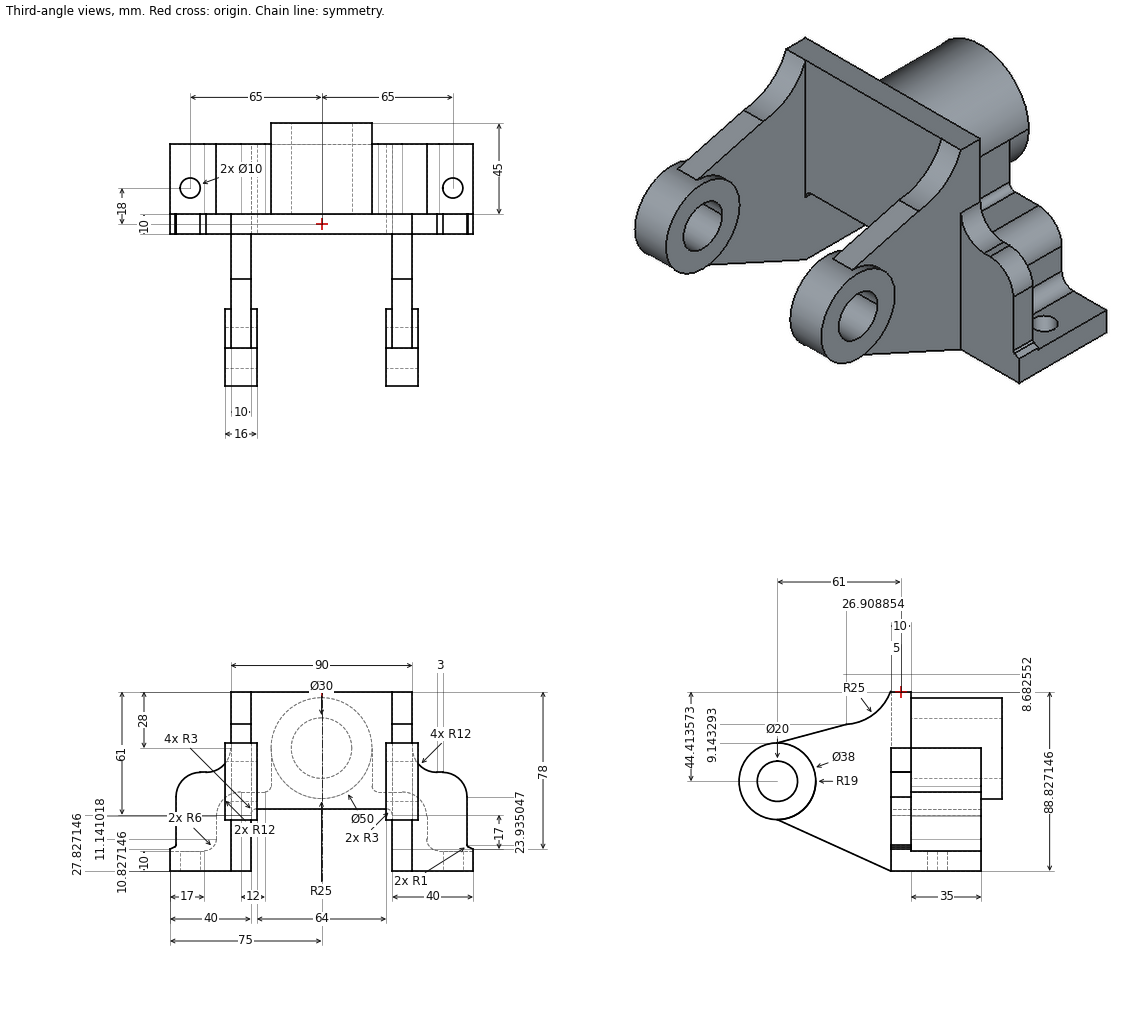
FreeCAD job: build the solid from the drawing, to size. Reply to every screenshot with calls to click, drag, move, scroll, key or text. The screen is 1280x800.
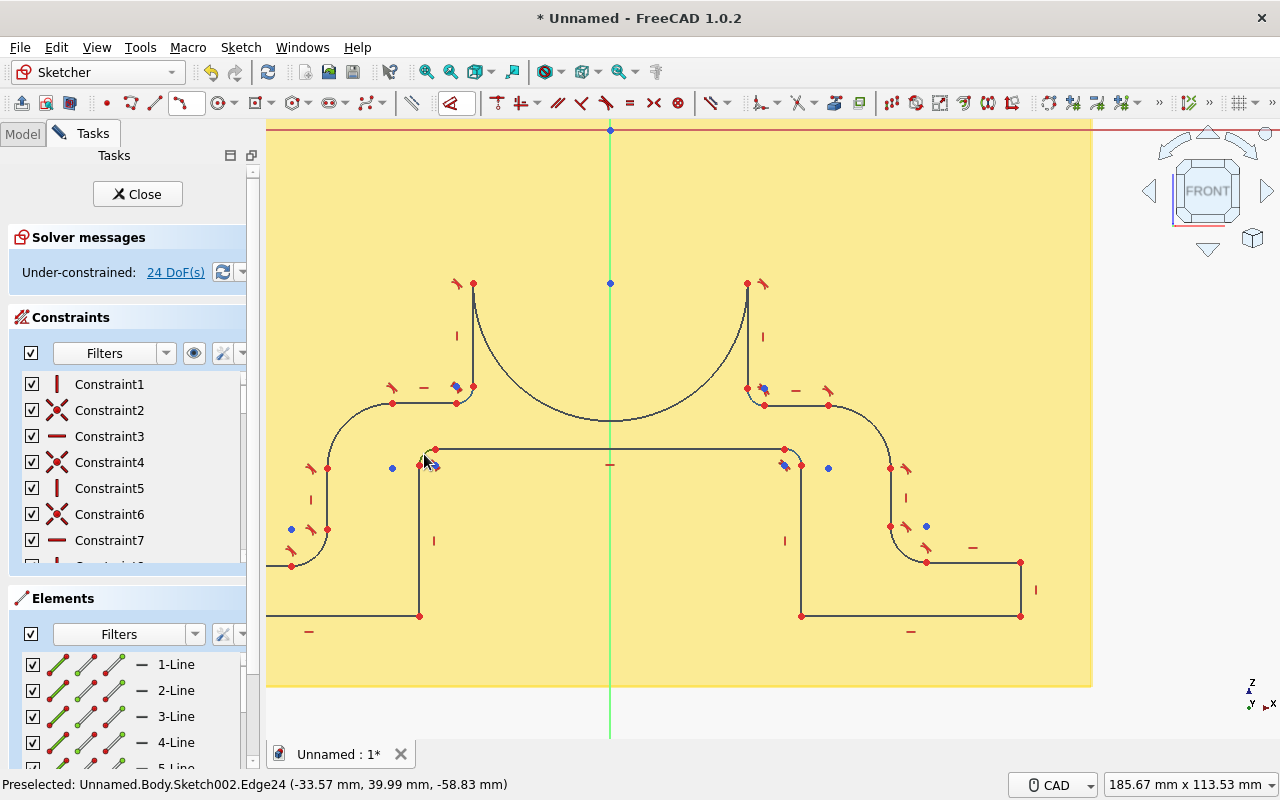
key(e)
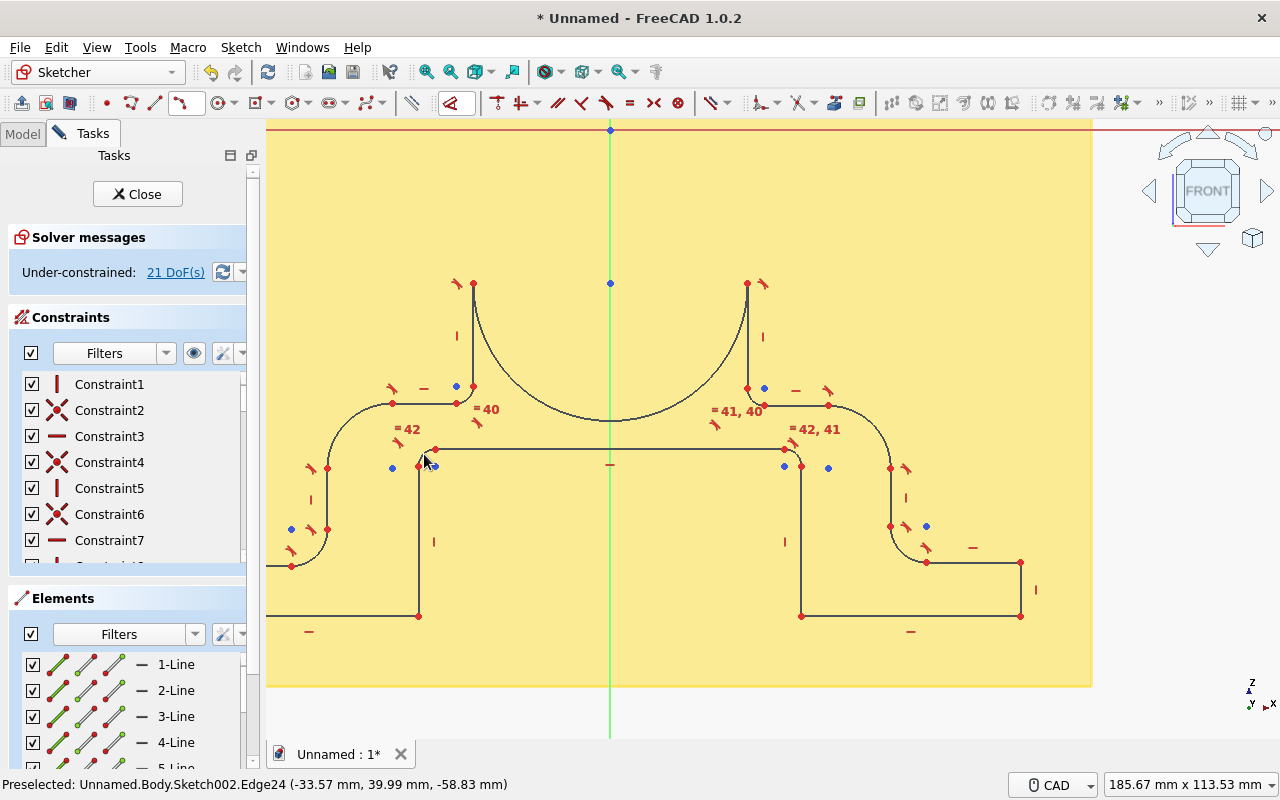
click(363, 411)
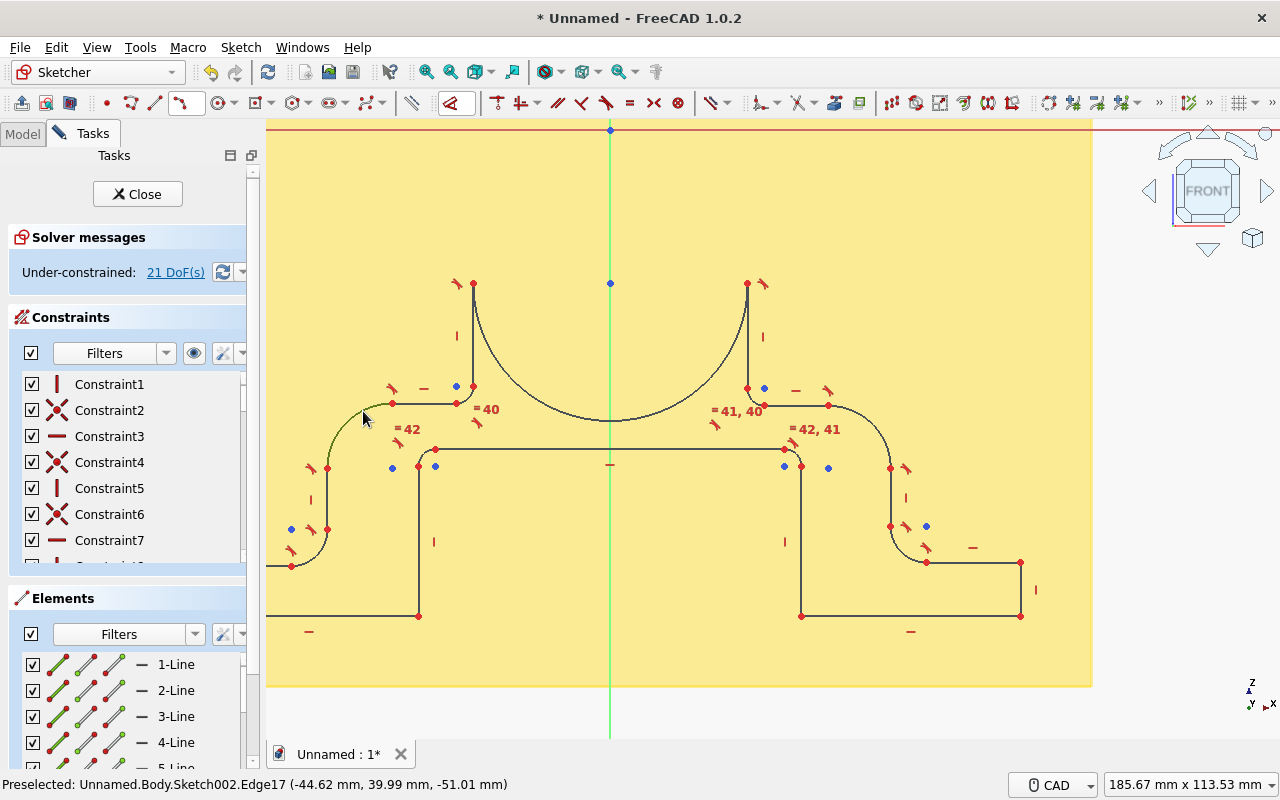
click(884, 440)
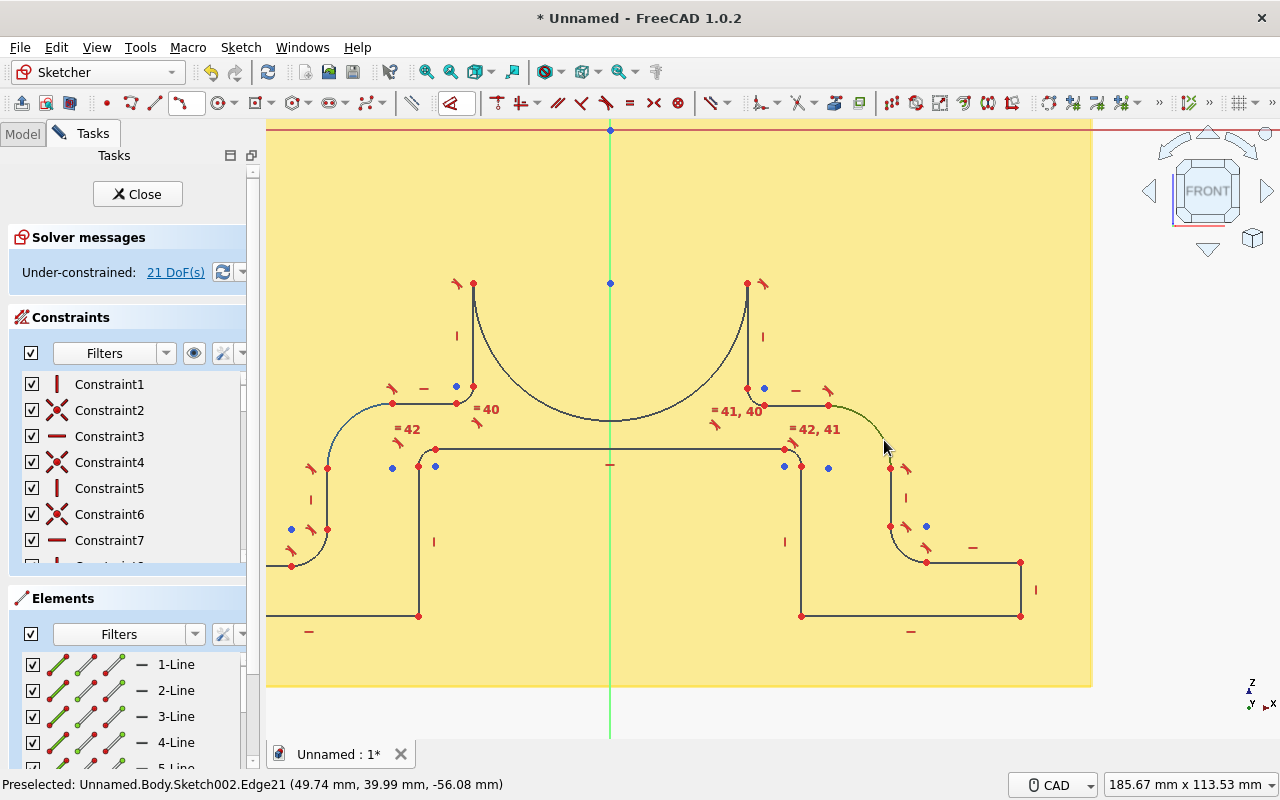
key(e)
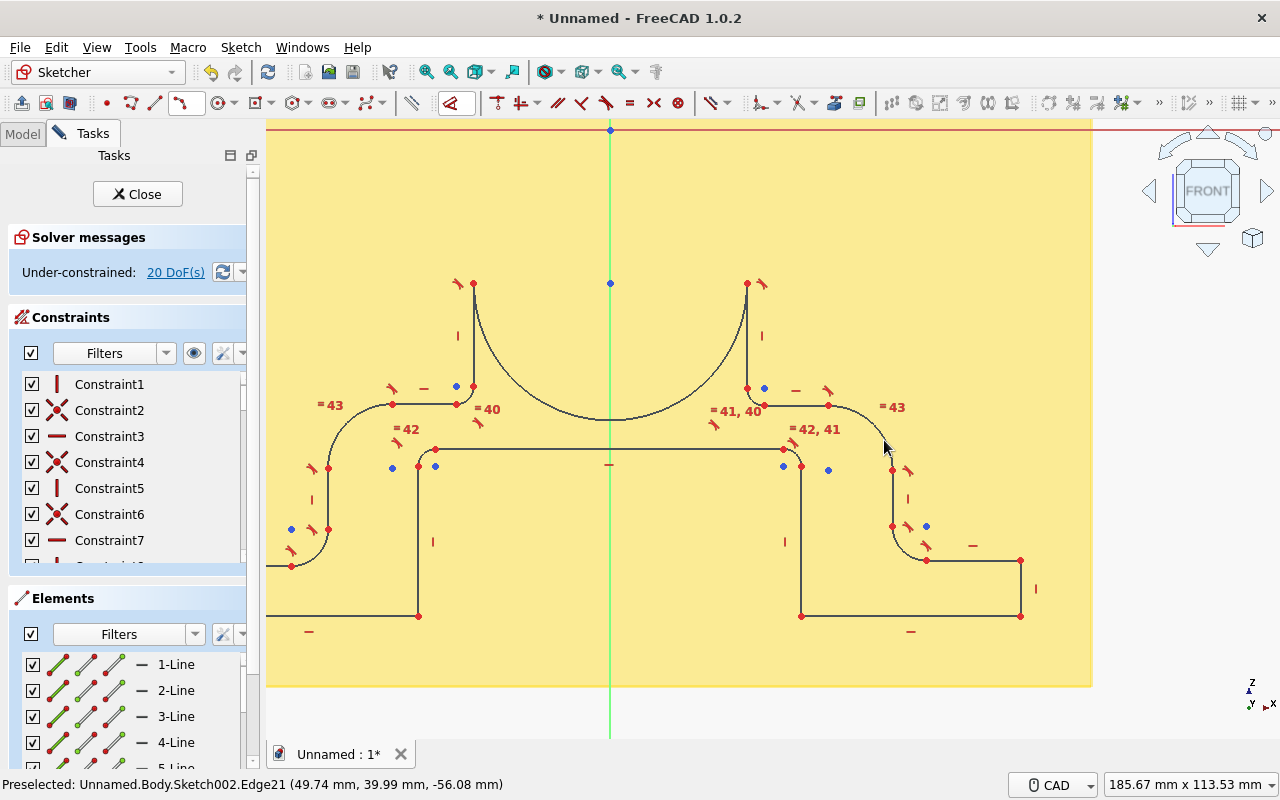
click(308, 562)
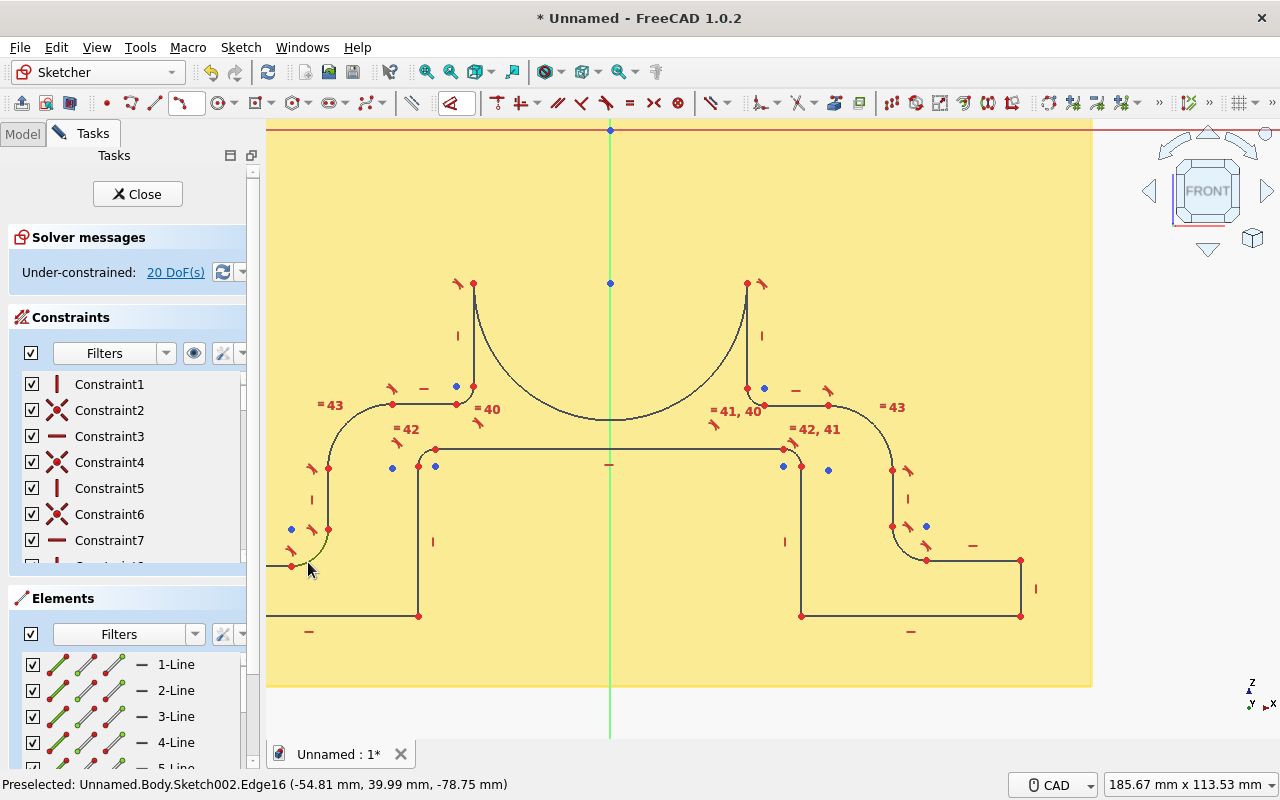
click(896, 542)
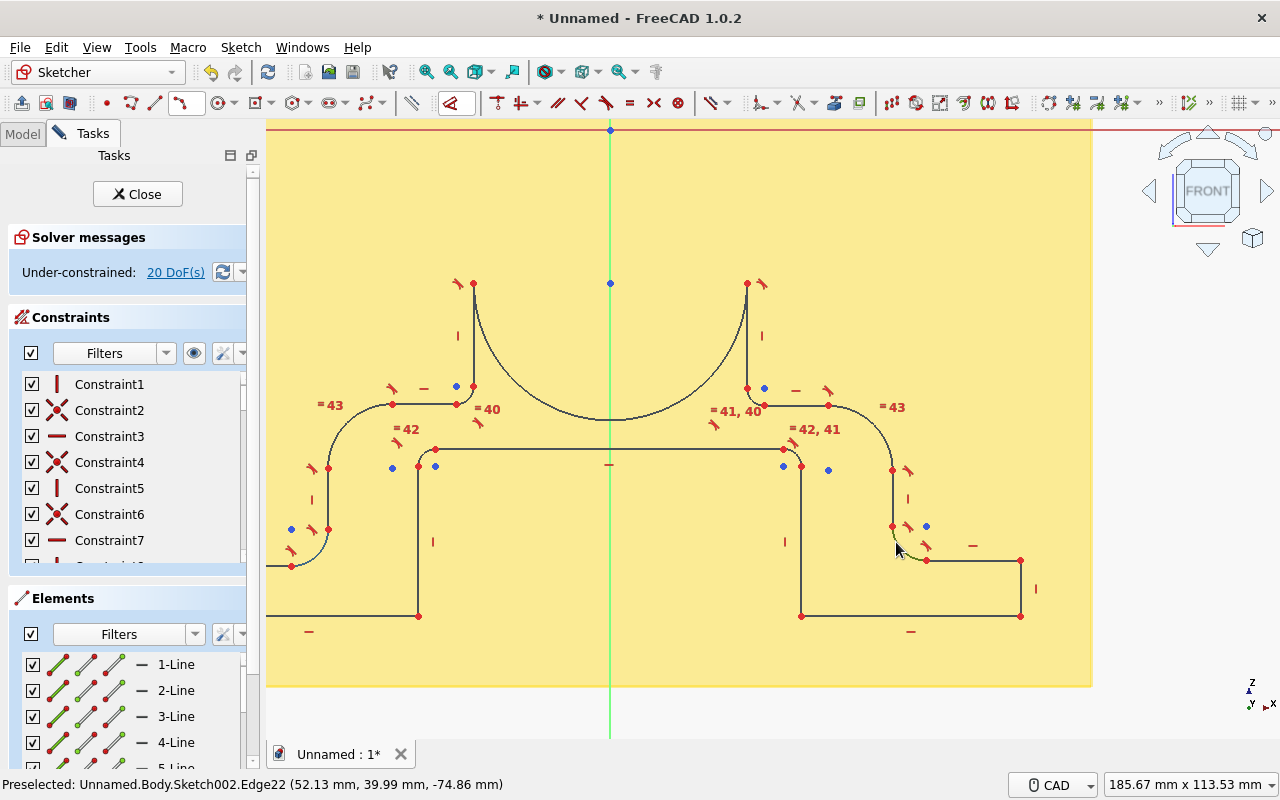
click(630, 104)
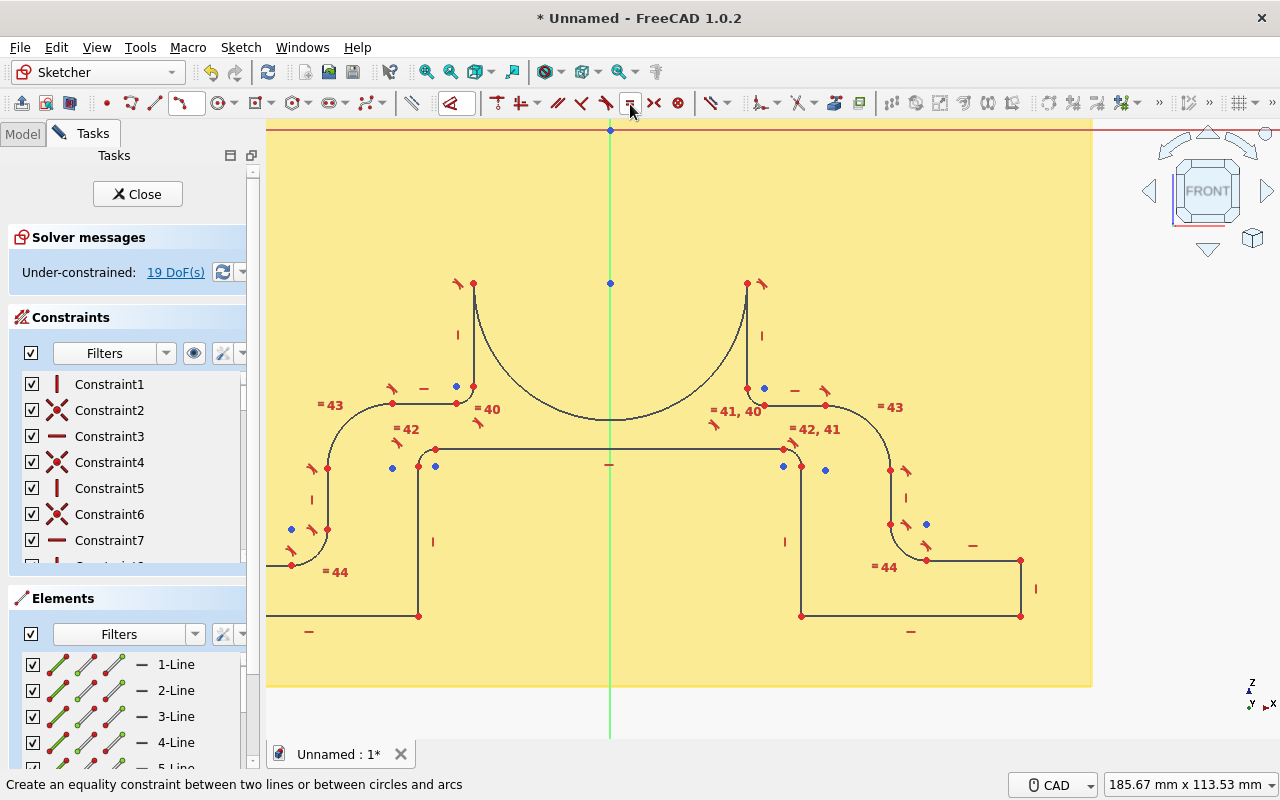
click(611, 284)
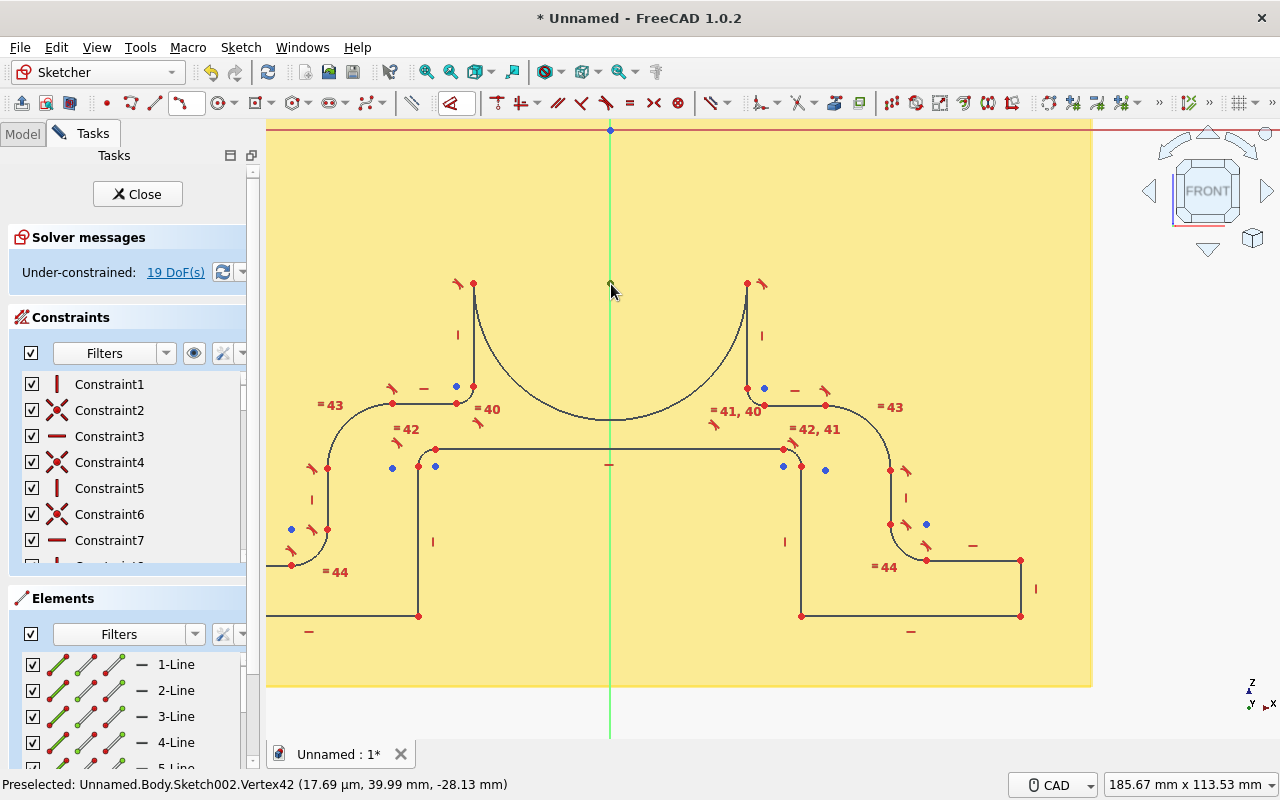
click(610, 671)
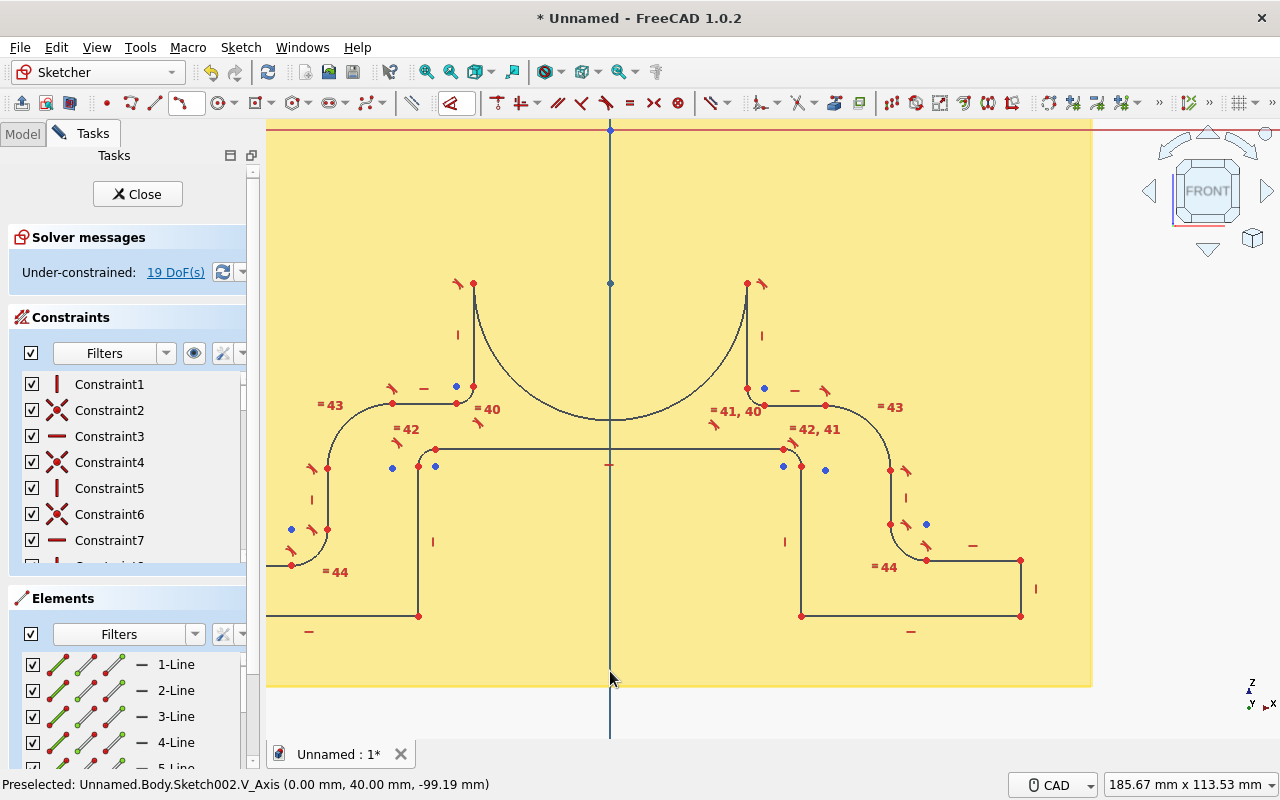
key(c)